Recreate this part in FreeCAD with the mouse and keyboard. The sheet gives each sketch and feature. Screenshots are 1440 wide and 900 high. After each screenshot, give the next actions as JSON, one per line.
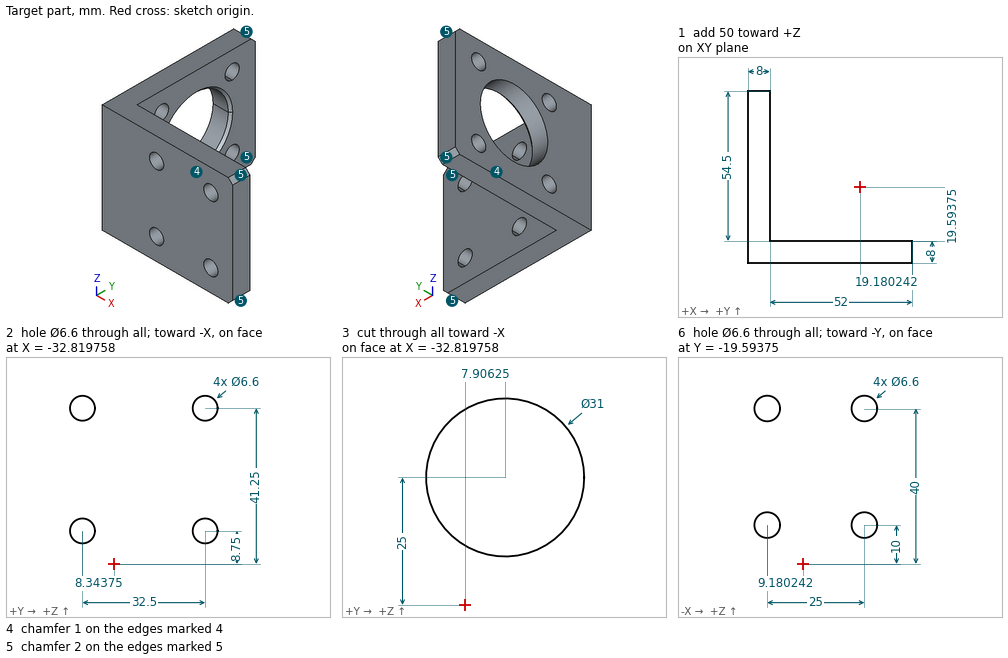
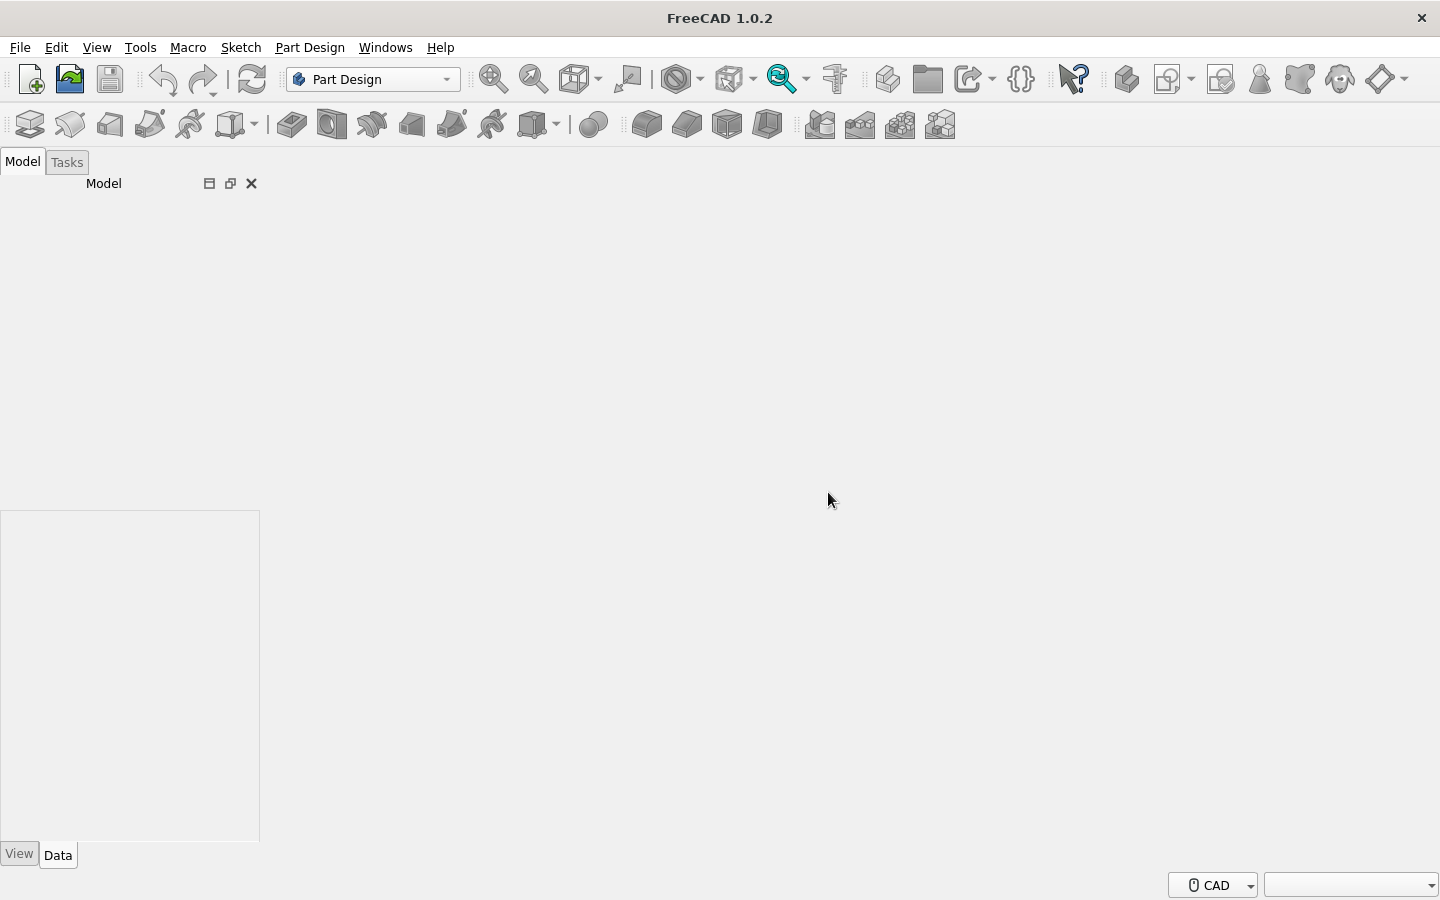
{"action": "left_click", "coordinate": [30, 80]}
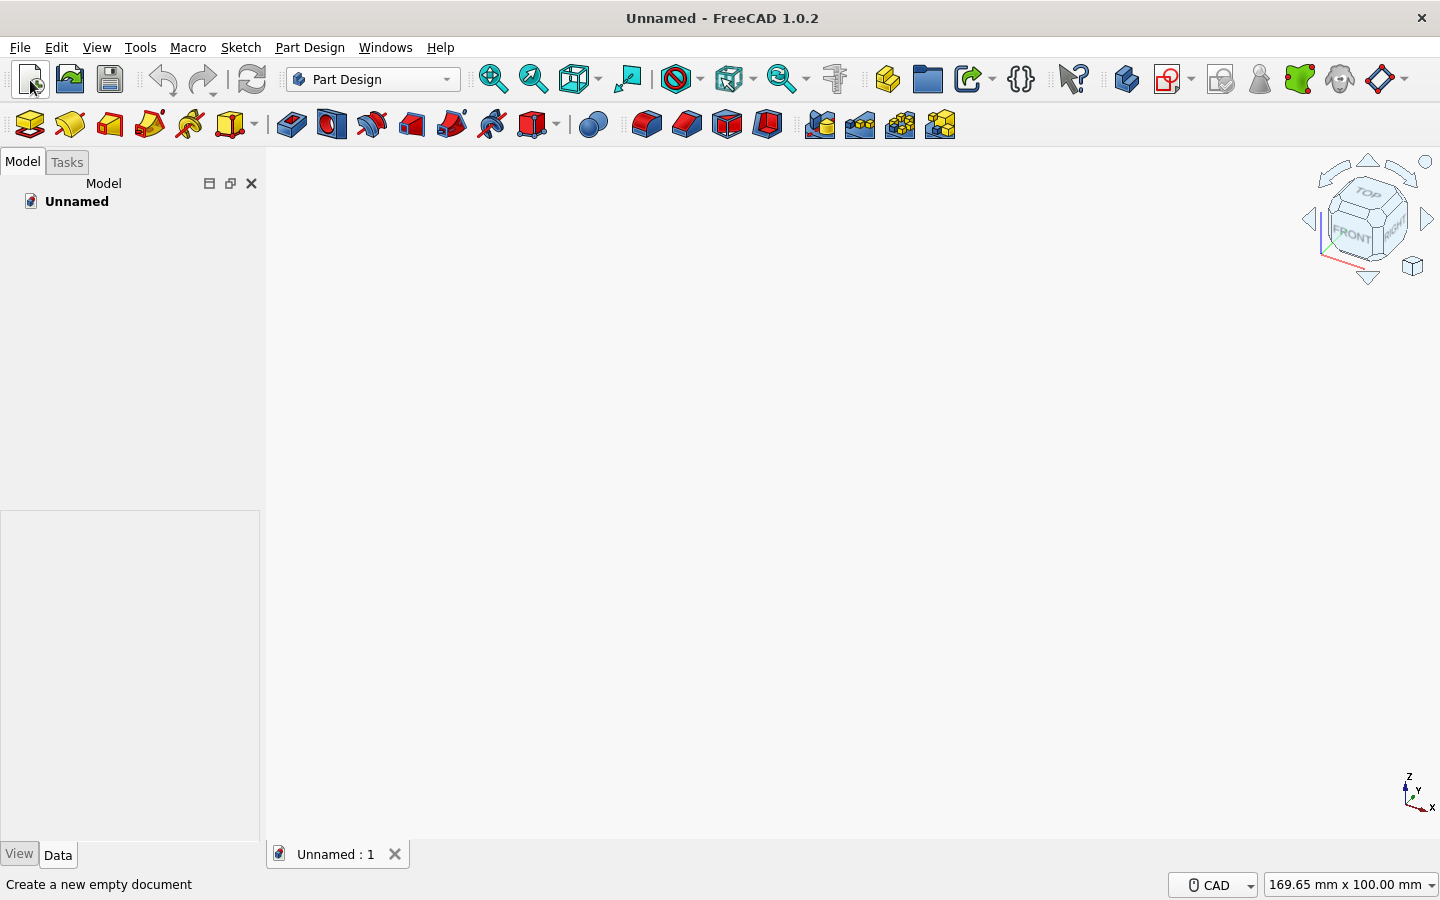
{"action": "left_click", "coordinate": [1168, 80]}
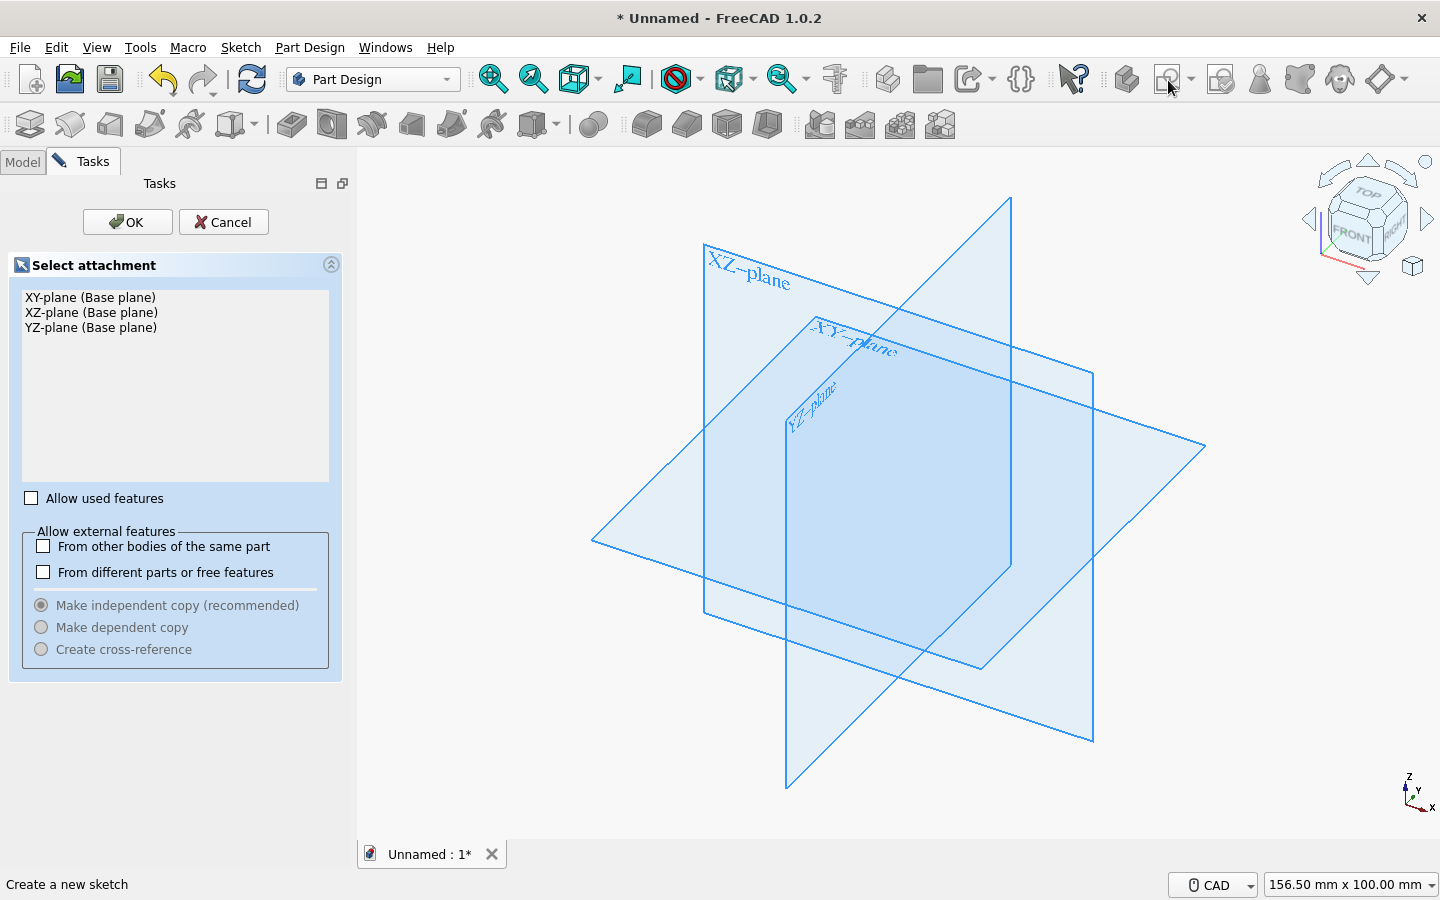
{"action": "left_click", "coordinate": [82, 298]}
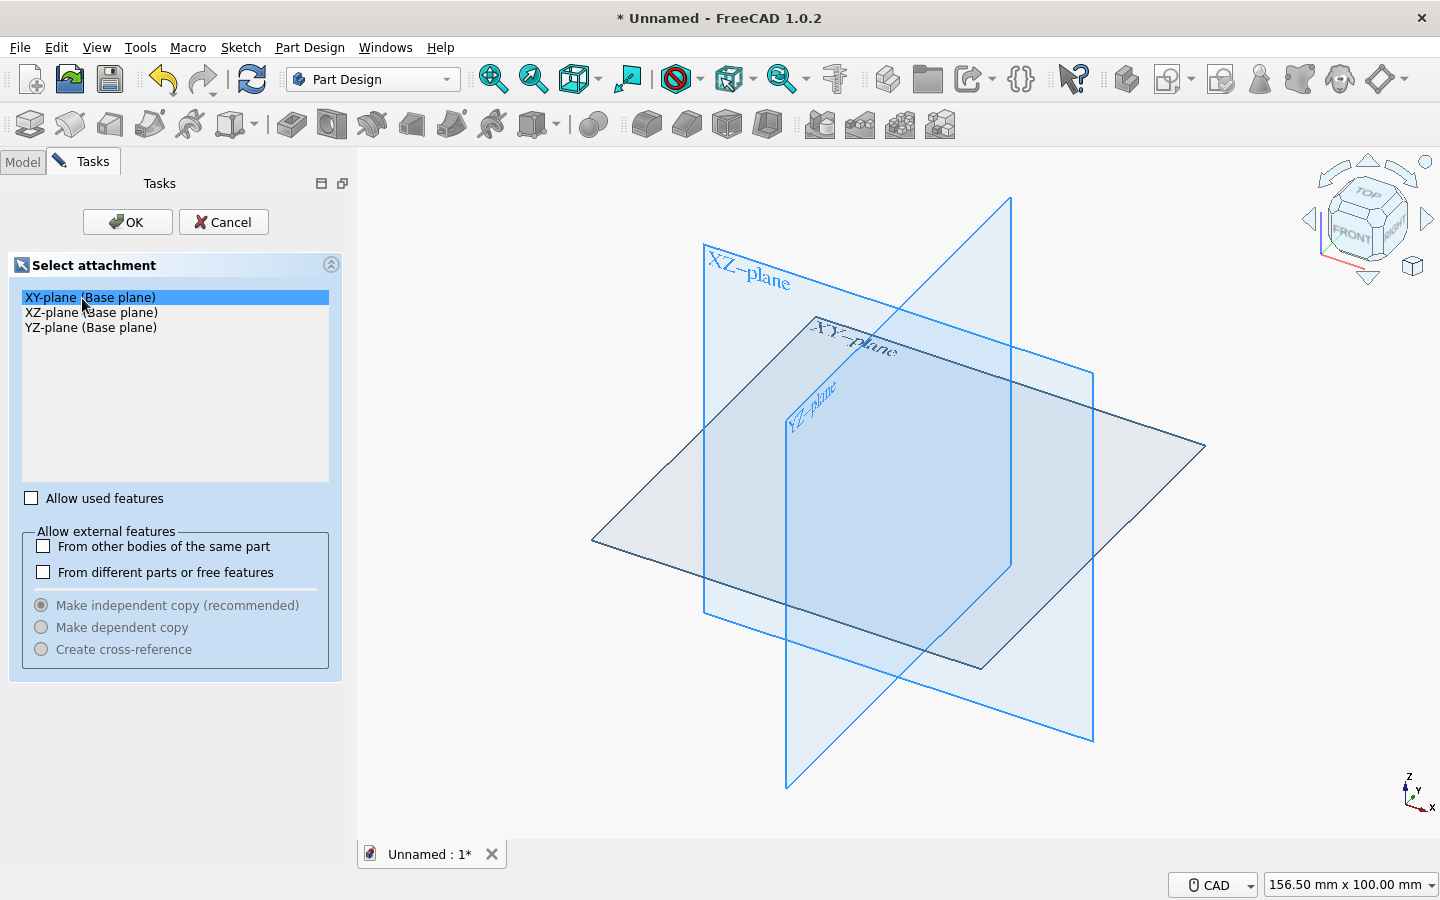
{"action": "left_click", "coordinate": [128, 222]}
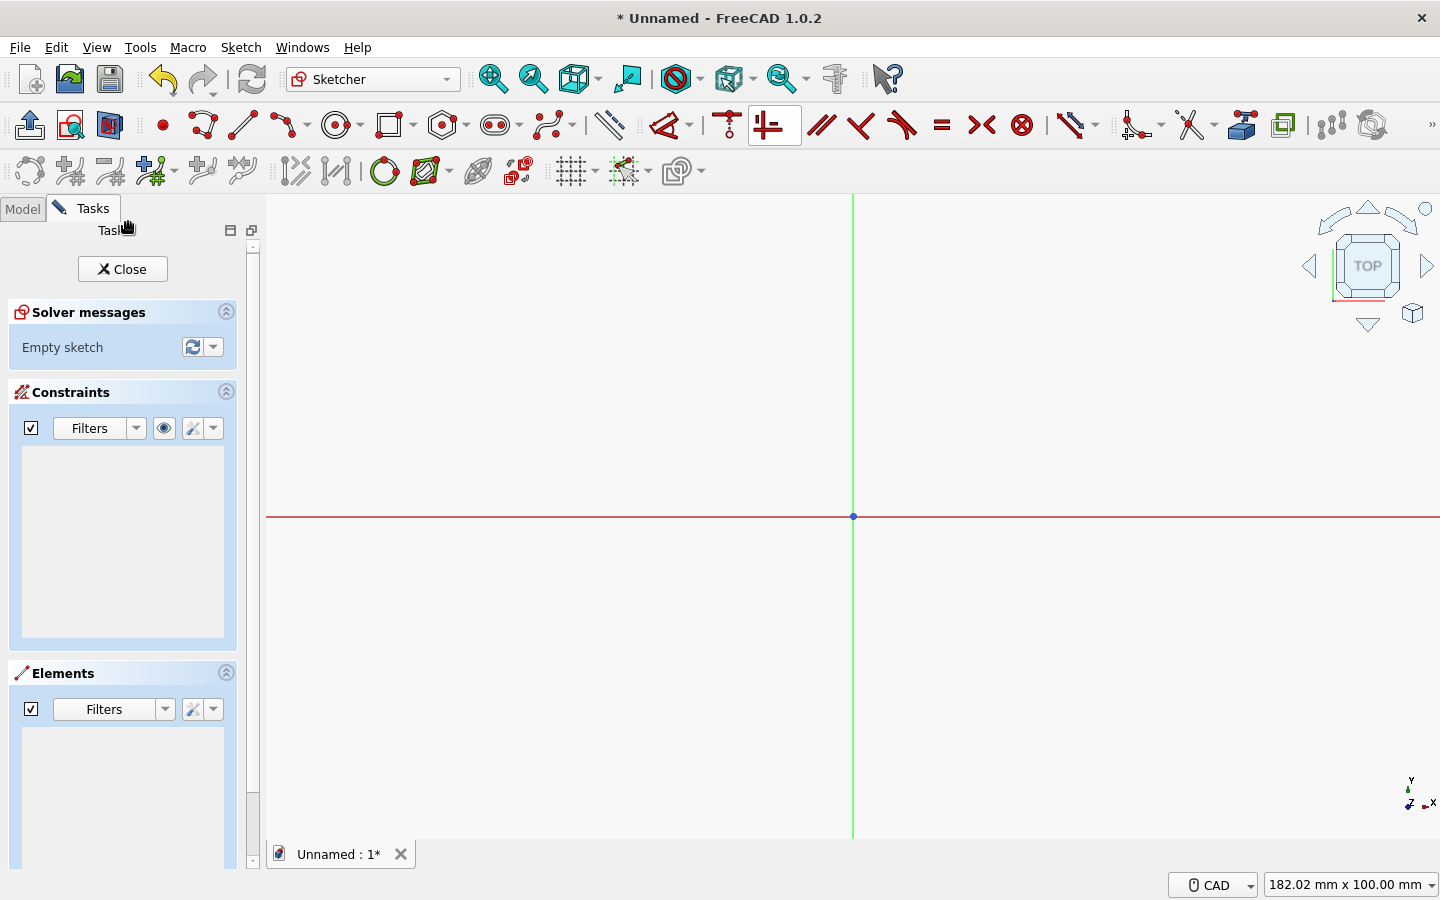
{"action": "left_click", "coordinate": [204, 126]}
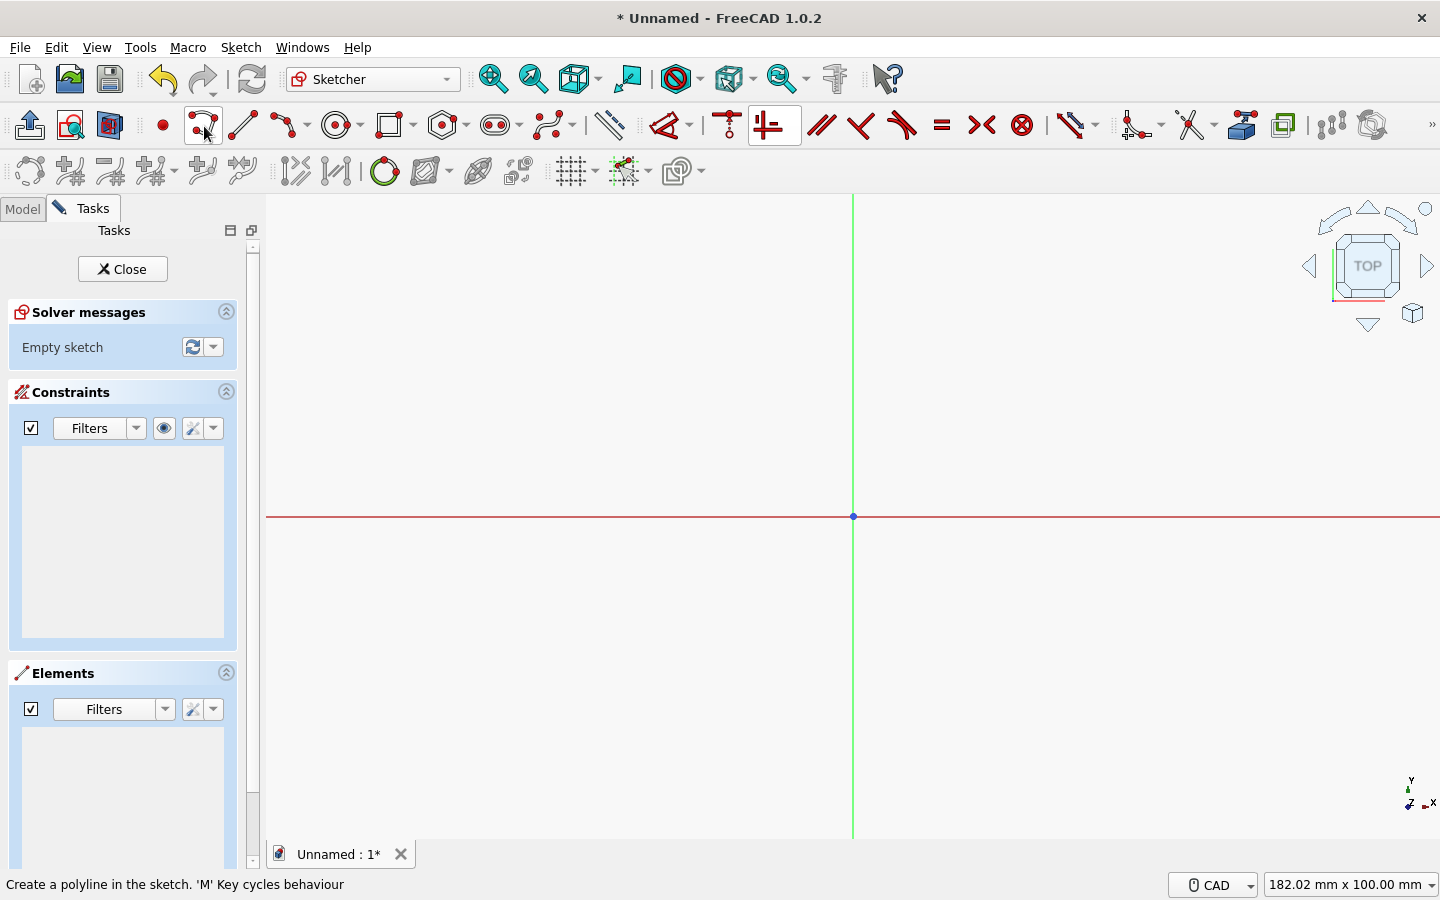
{"action": "left_click", "coordinate": [977, 643]}
{"action": "left_click", "coordinate": [641, 643]}
{"action": "left_click", "coordinate": [641, 291]}
{"action": "left_click", "coordinate": [590, 291]}
{"action": "left_click", "coordinate": [590, 694]}
{"action": "left_click", "coordinate": [977, 694]}
{"action": "left_click", "coordinate": [977, 644]}
{"action": "key", "text": "Escape"}
{"action": "key", "text": "Escape"}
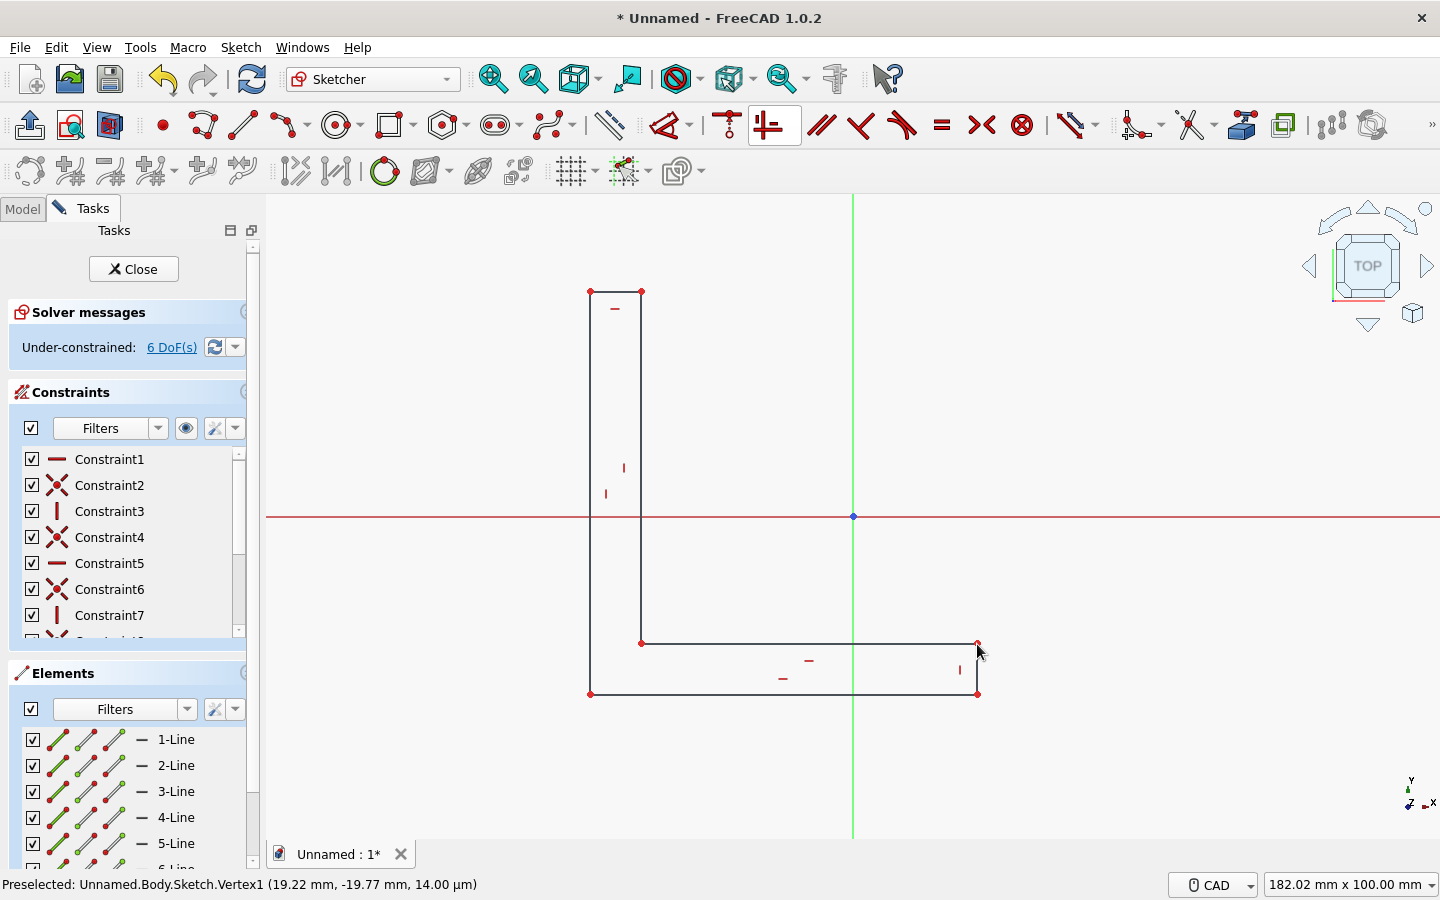
{"action": "left_click", "coordinate": [664, 126]}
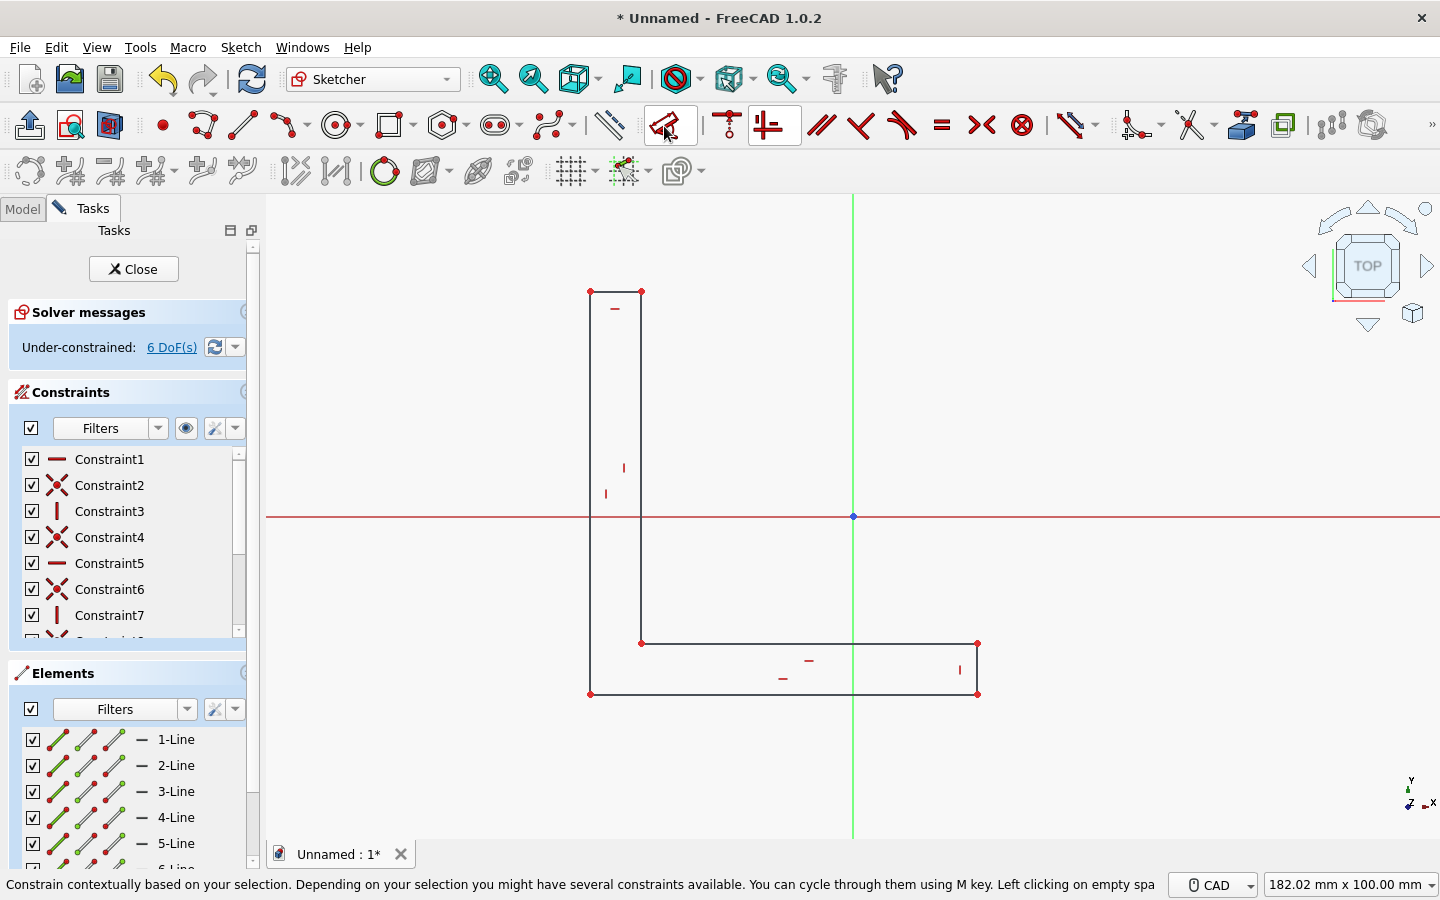
{"action": "left_click", "coordinate": [626, 292]}
{"action": "left_click", "coordinate": [616, 258]}